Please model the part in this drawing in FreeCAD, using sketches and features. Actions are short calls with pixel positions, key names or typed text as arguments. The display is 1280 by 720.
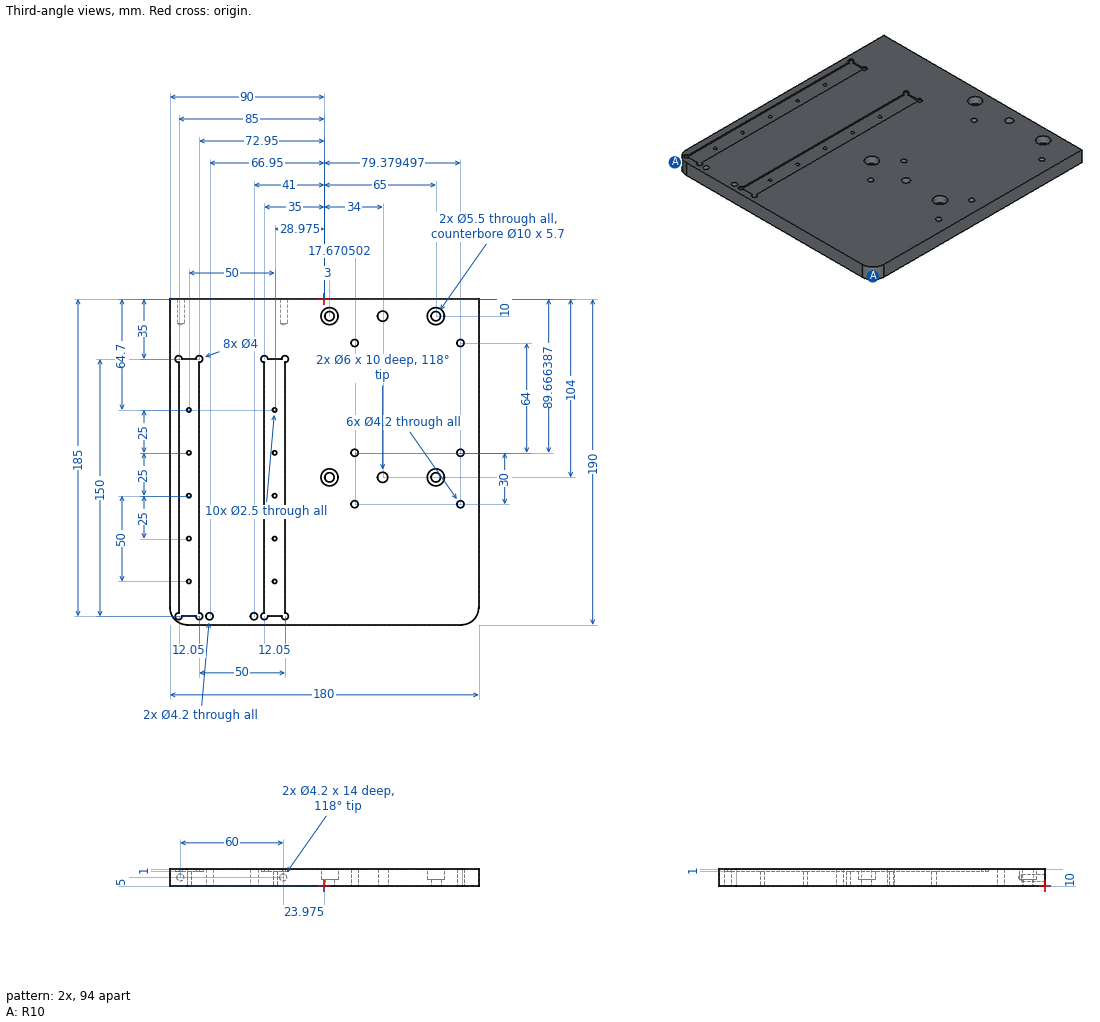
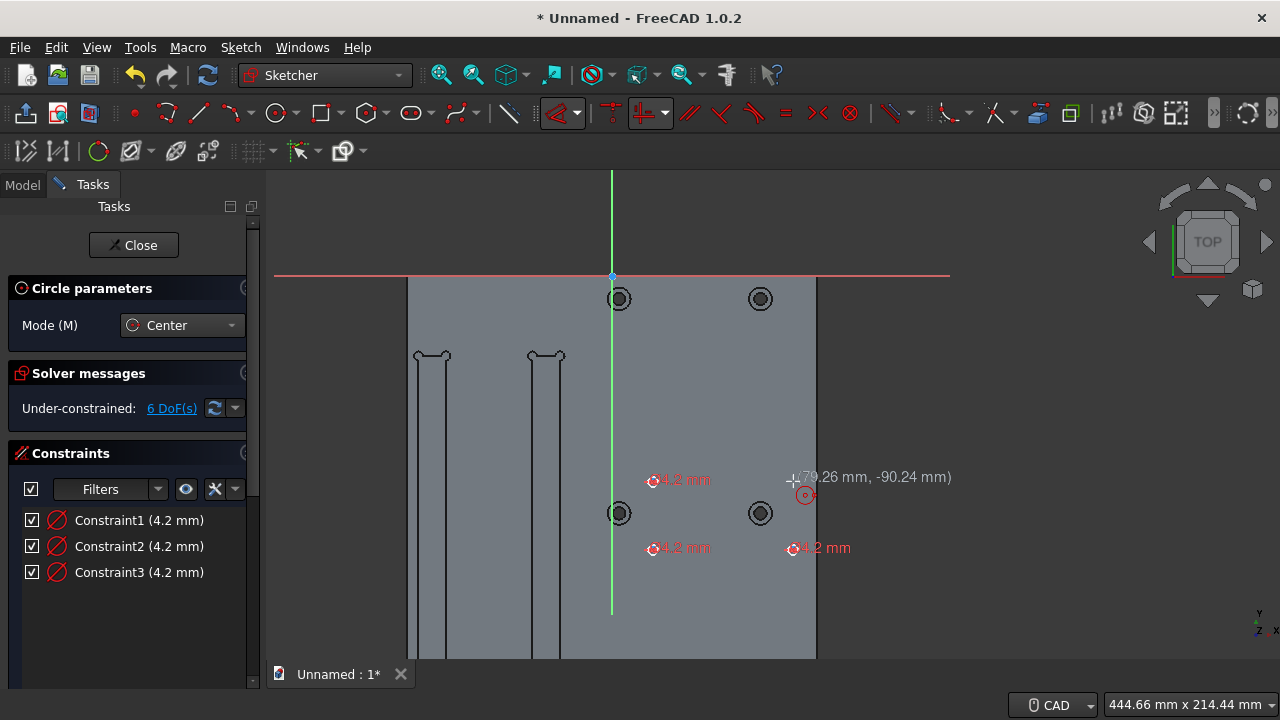
click(793, 481)
move(797, 477)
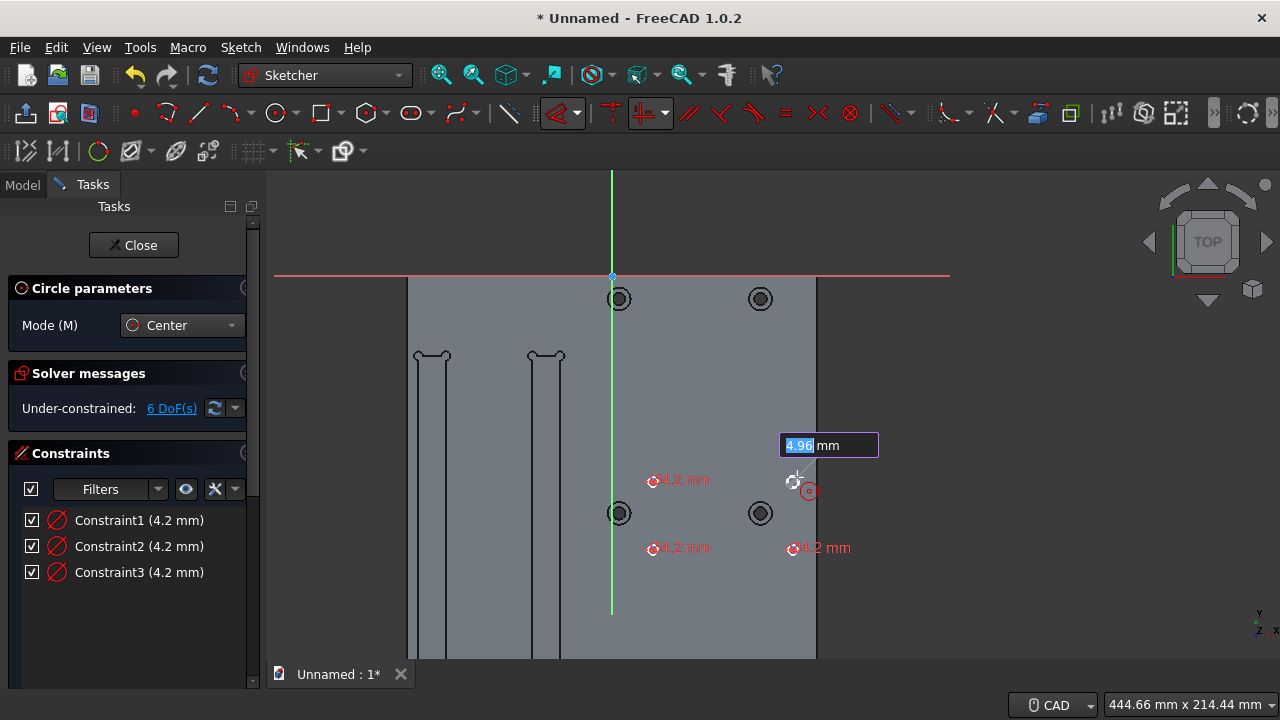
text(4.2)
key(Return)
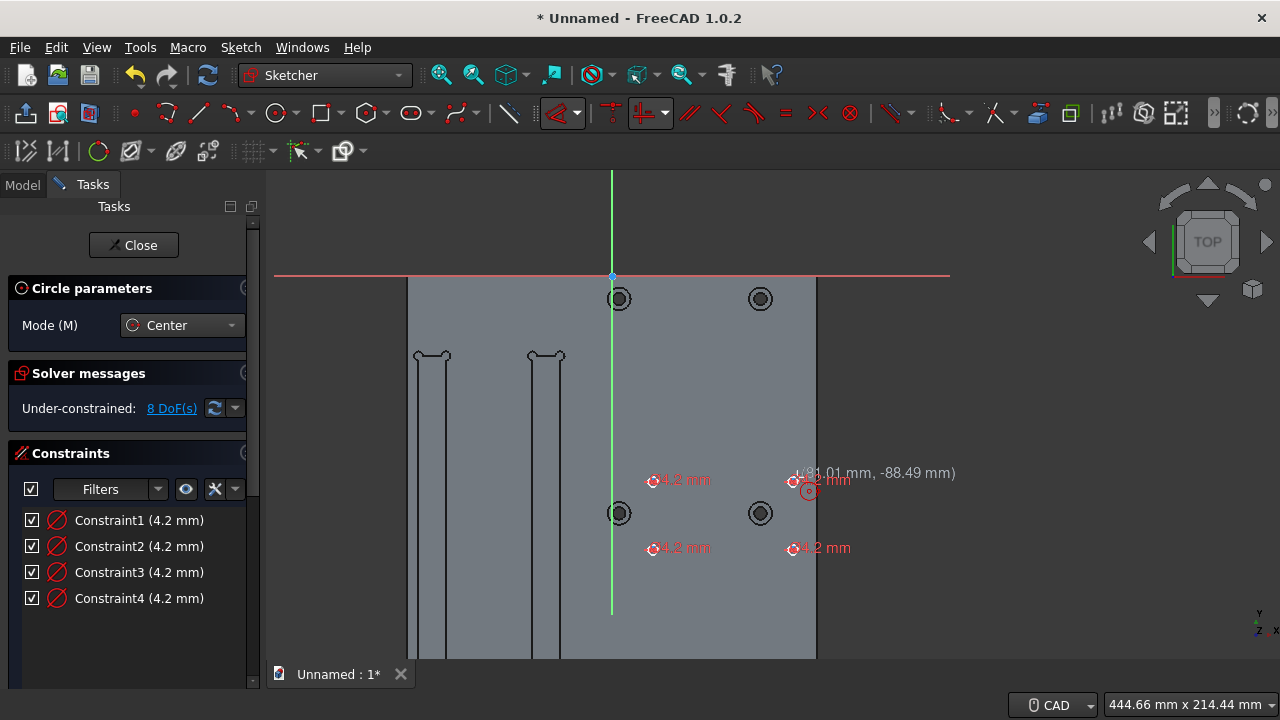
scroll(793, 335, up, 8)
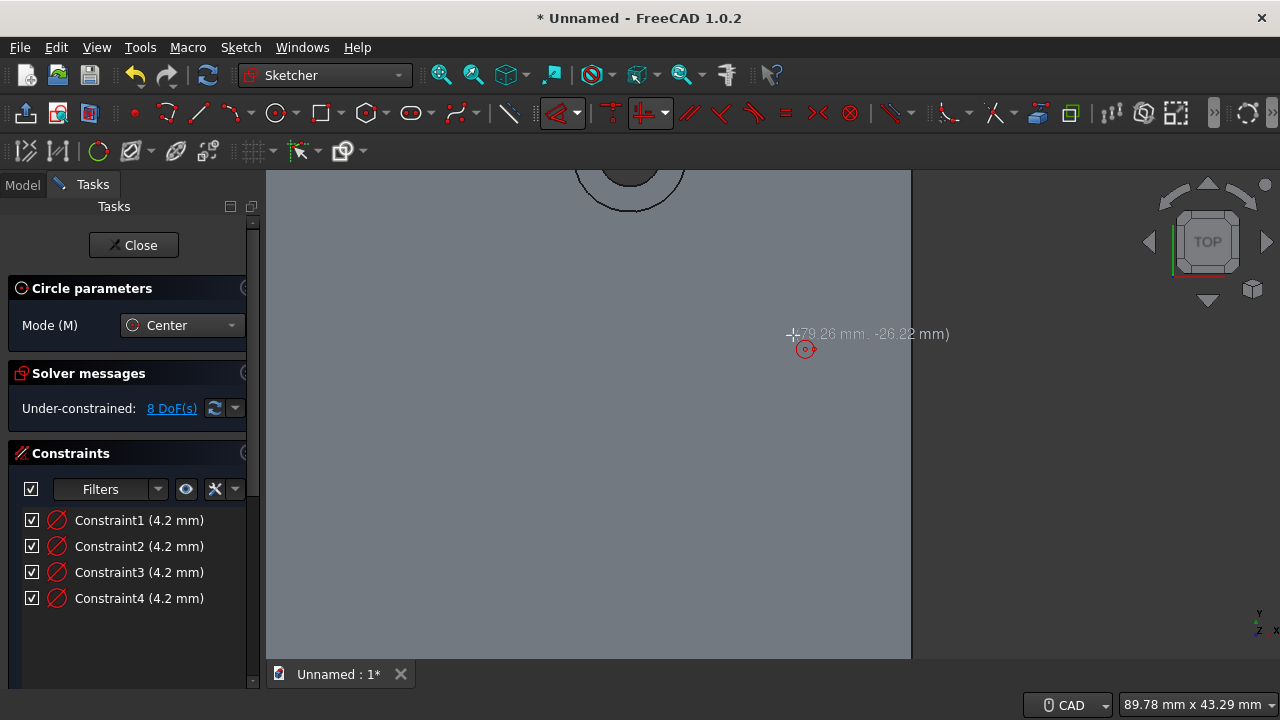
scroll(793, 335, down, 8)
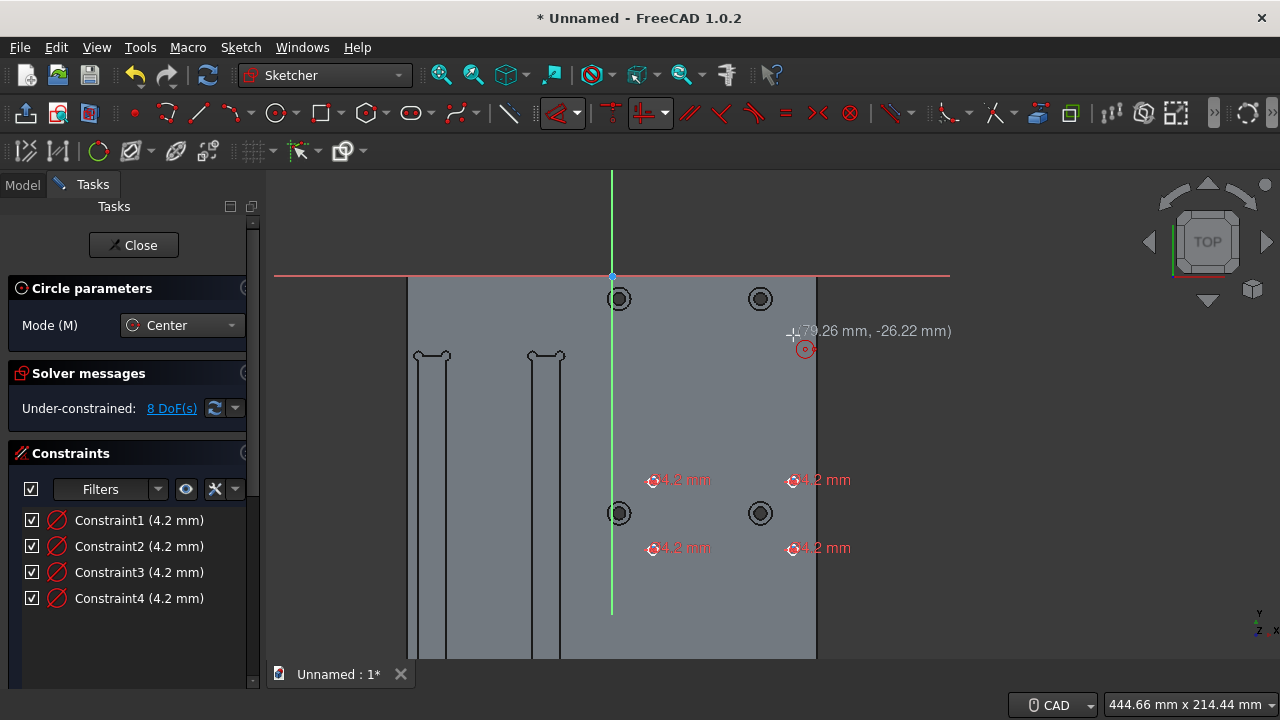
click(793, 335)
move(797, 331)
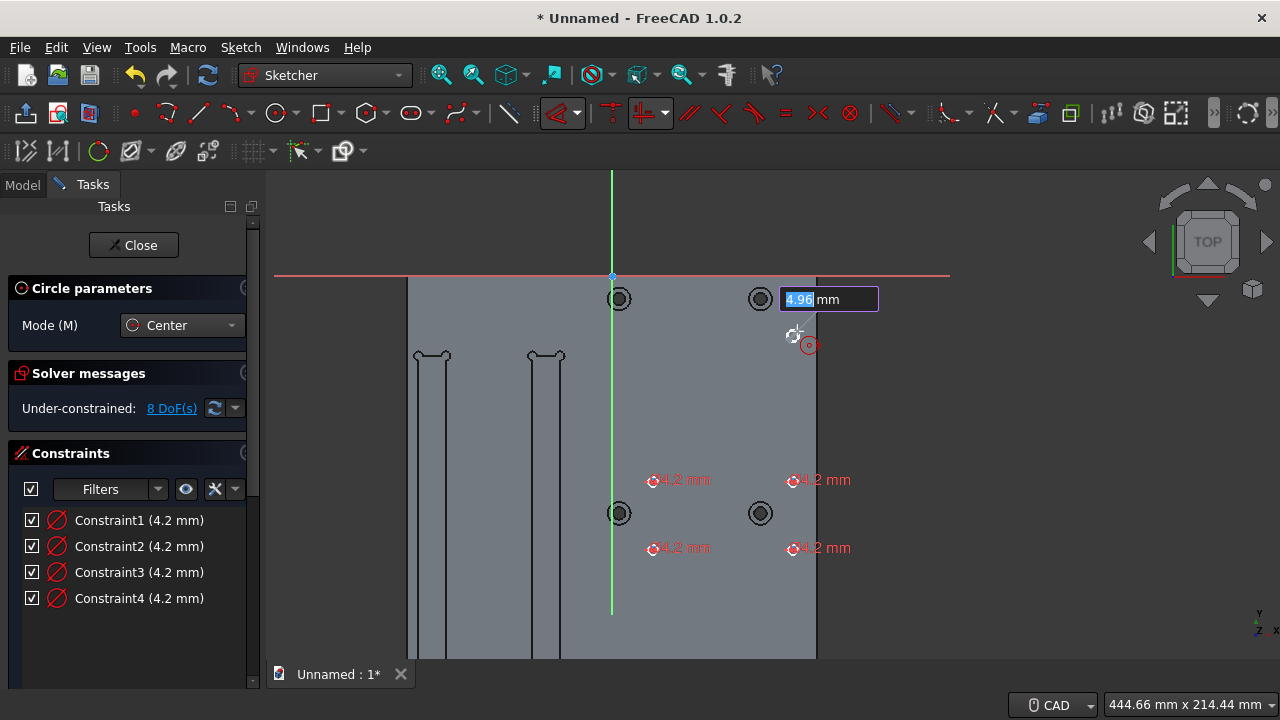
text(4.2)
key(Return)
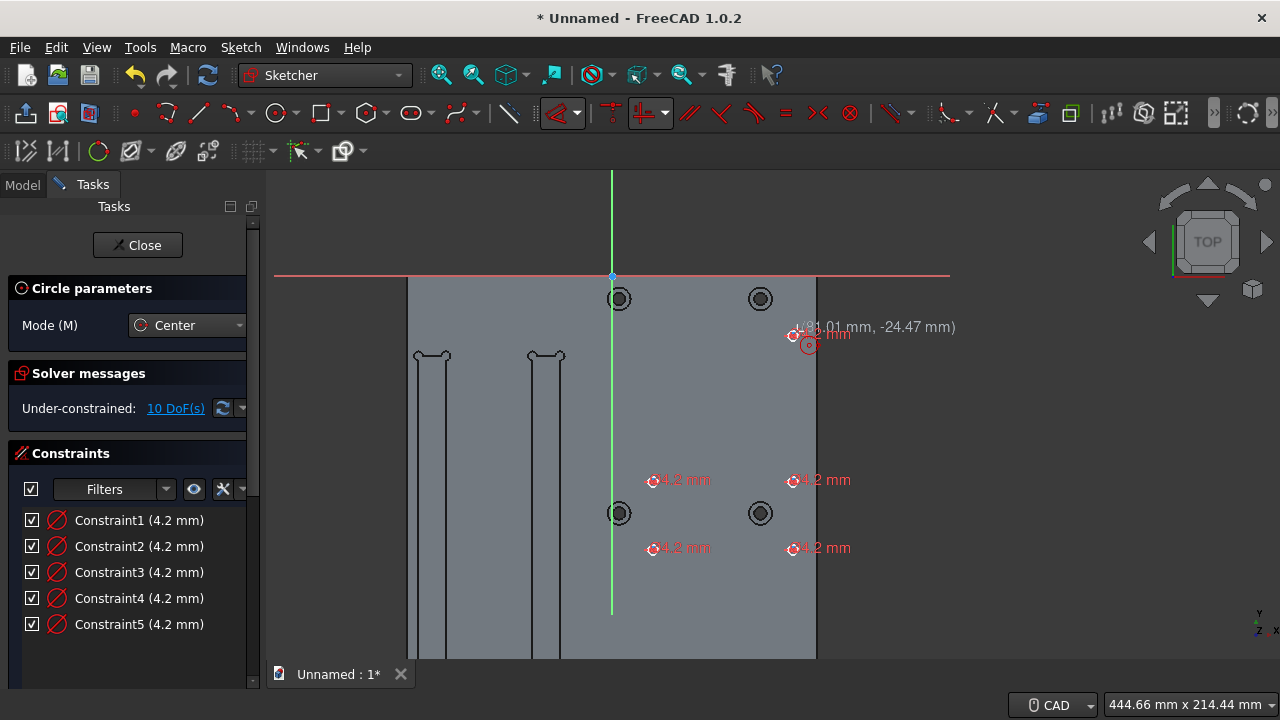
scroll(653, 335, up, 8)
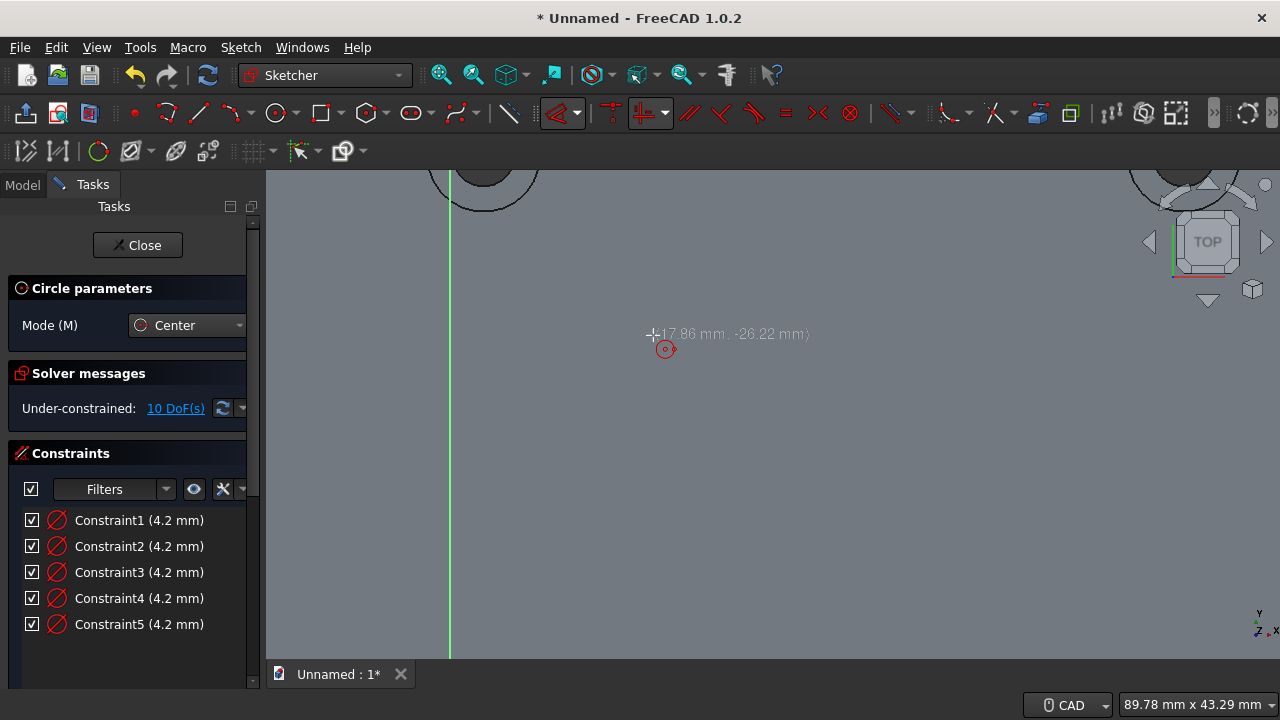
scroll(653, 335, down, 8)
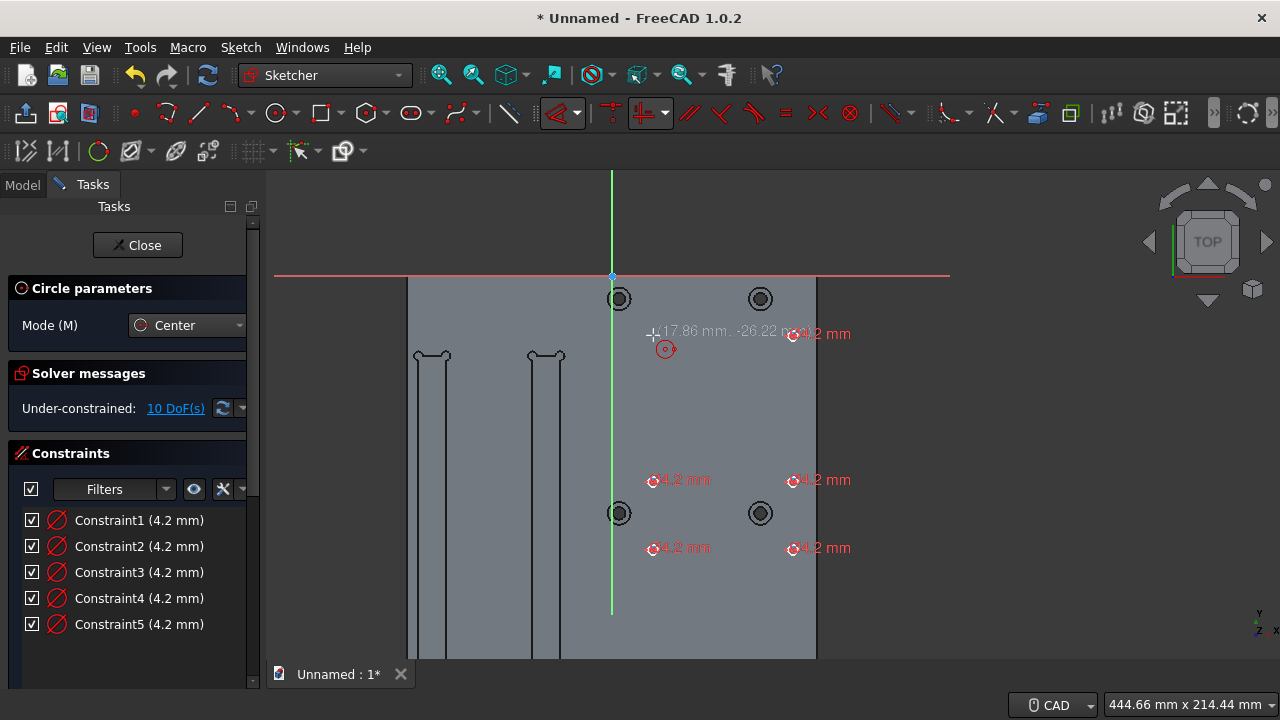
click(653, 335)
move(656, 331)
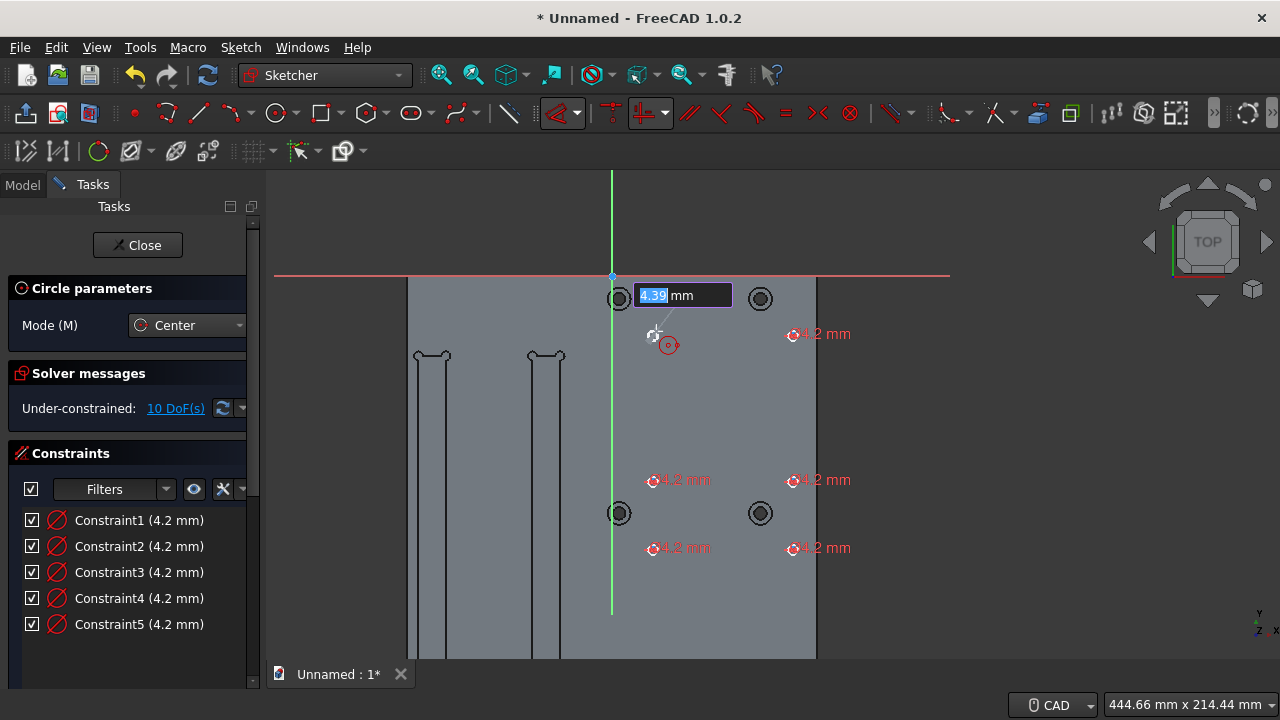
text(4.2)
key(Return)
key(Escape)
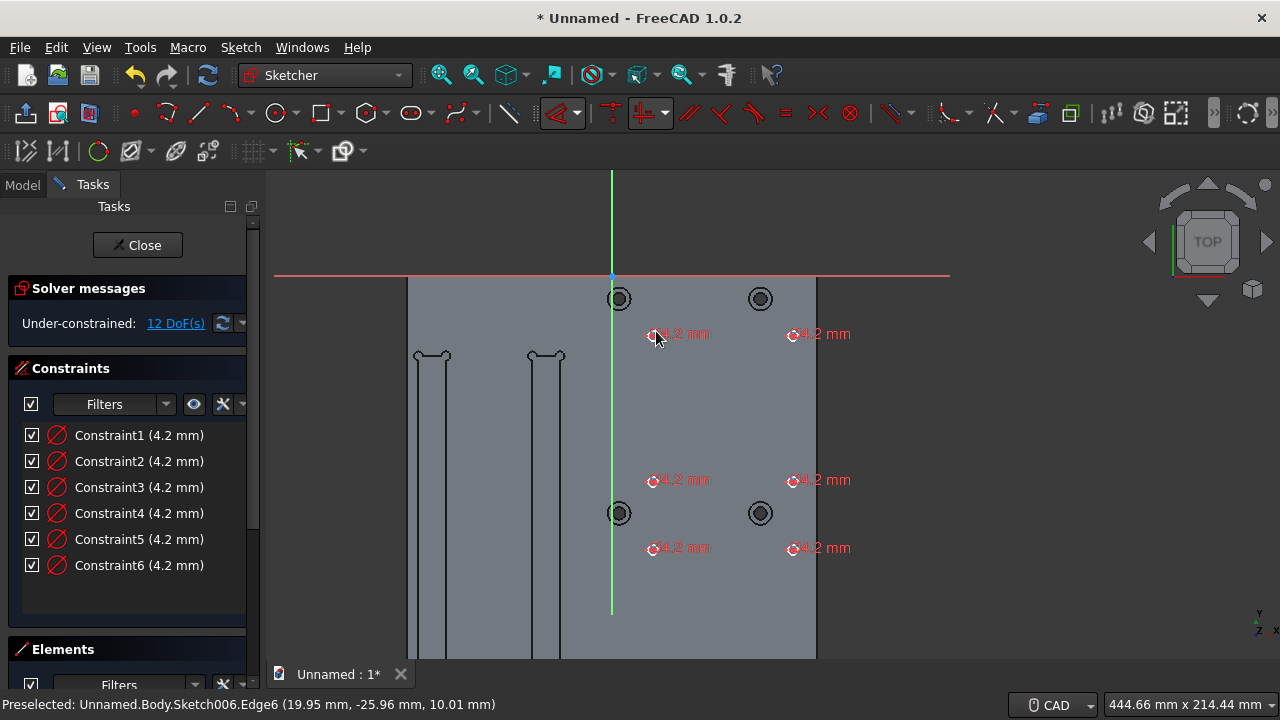
click(793, 550)